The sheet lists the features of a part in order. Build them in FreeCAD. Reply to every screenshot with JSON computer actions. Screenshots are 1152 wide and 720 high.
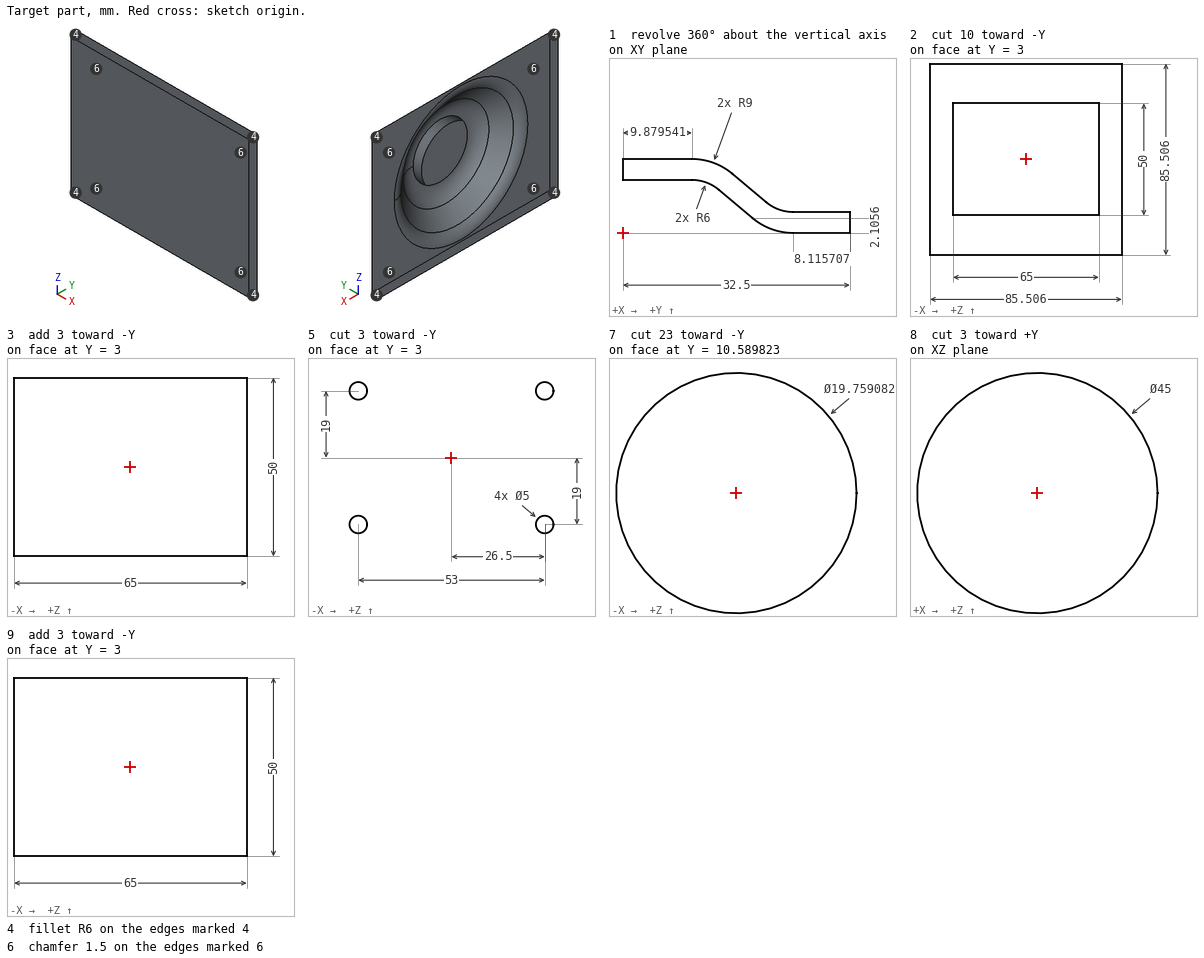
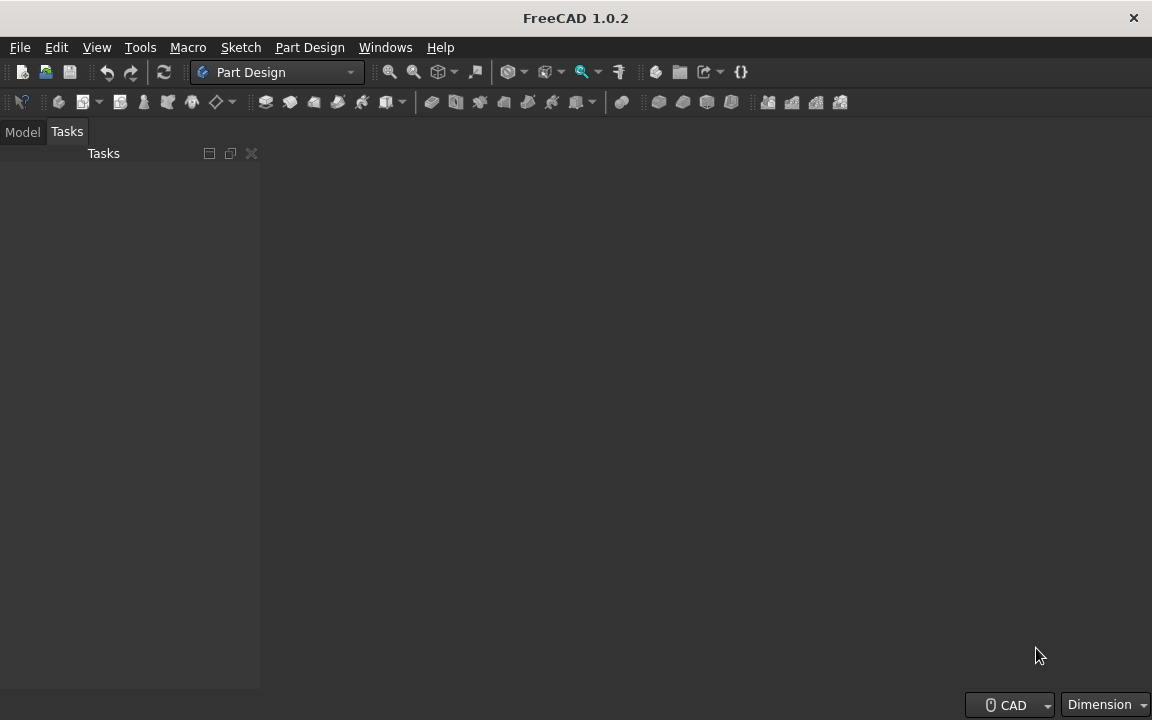
{"action": "left_click", "coordinate": [22, 72]}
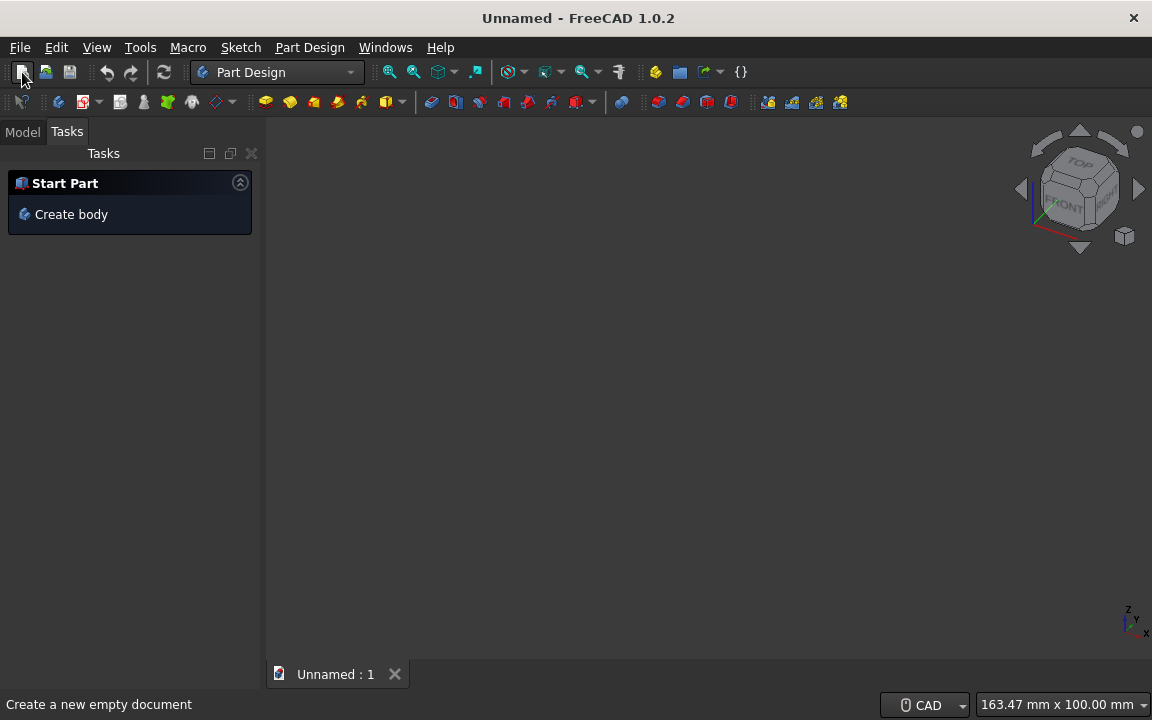
{"action": "left_click", "coordinate": [84, 102]}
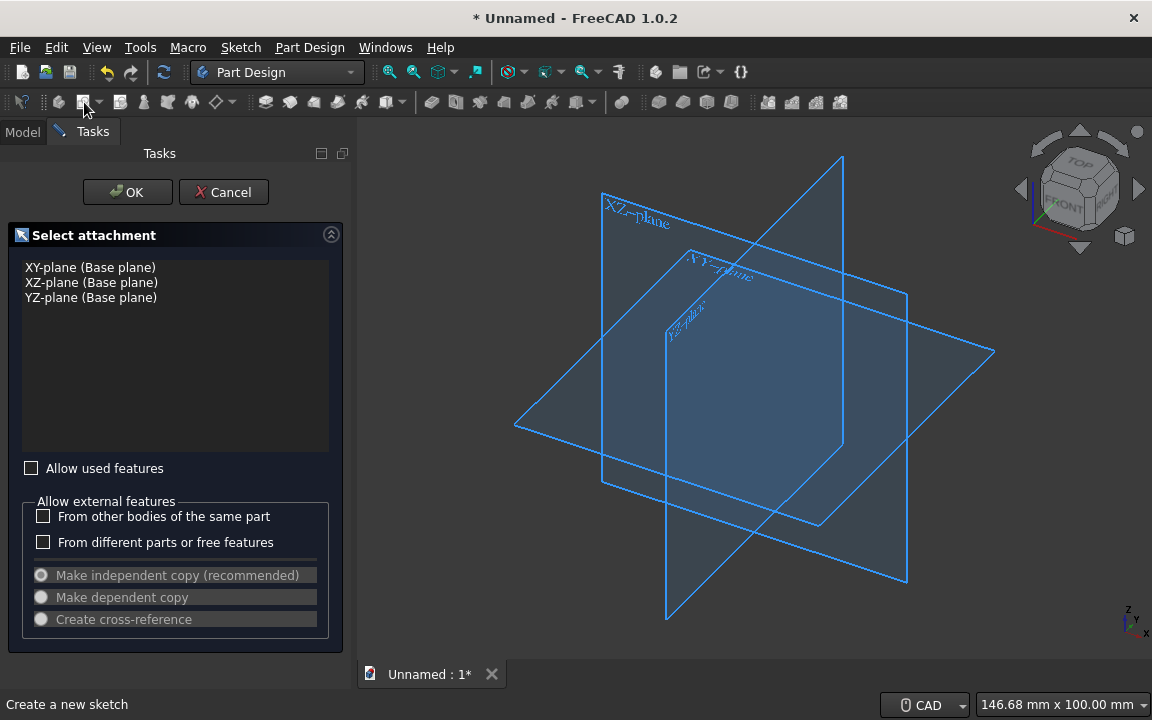
{"action": "left_click", "coordinate": [82, 268]}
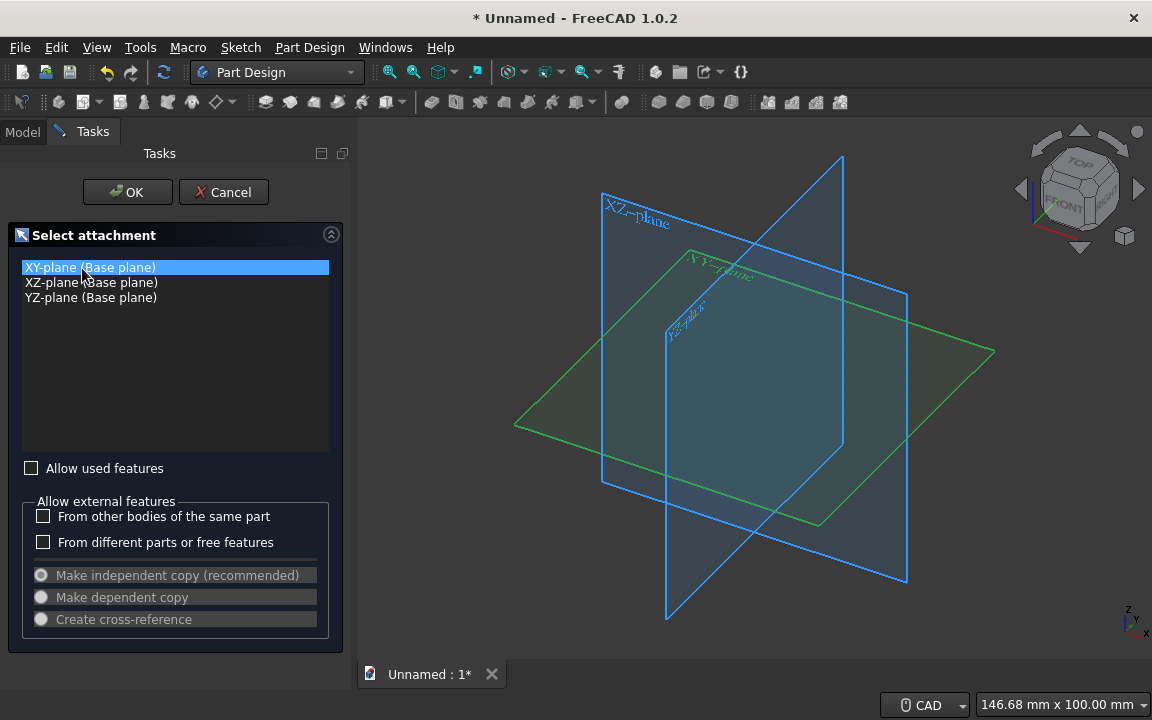
{"action": "left_click", "coordinate": [128, 192]}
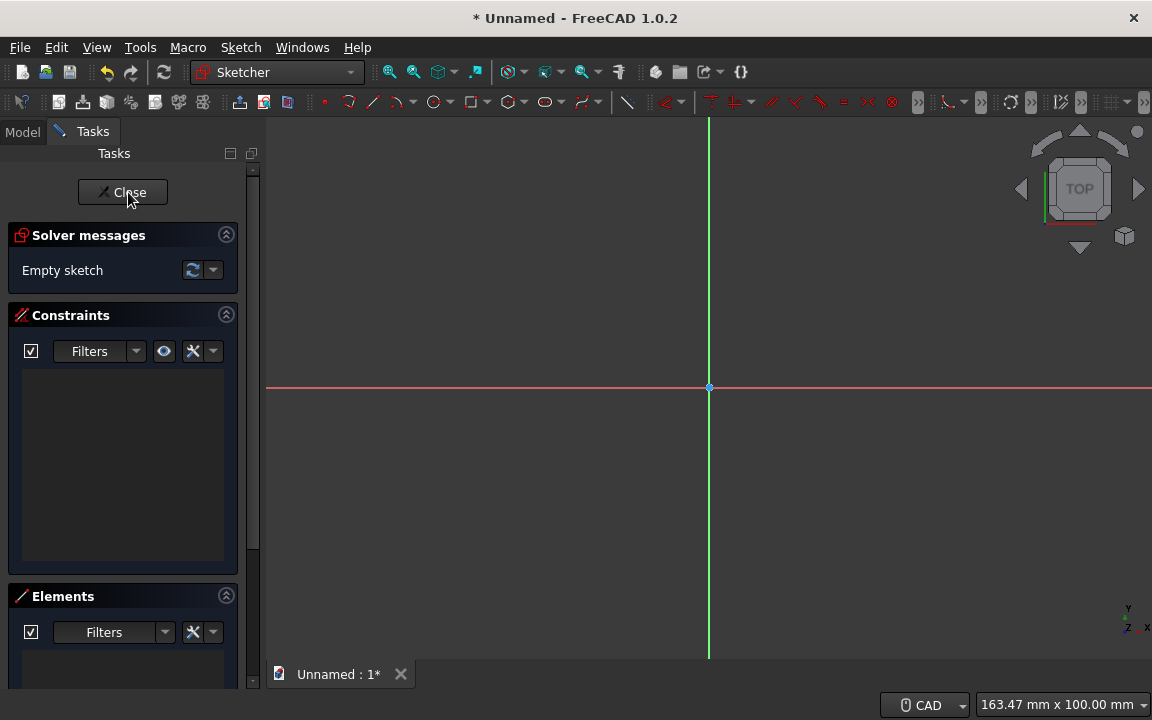
{"action": "scroll", "coordinate": [888, 343], "scroll_direction": "up", "scroll_amount": 5}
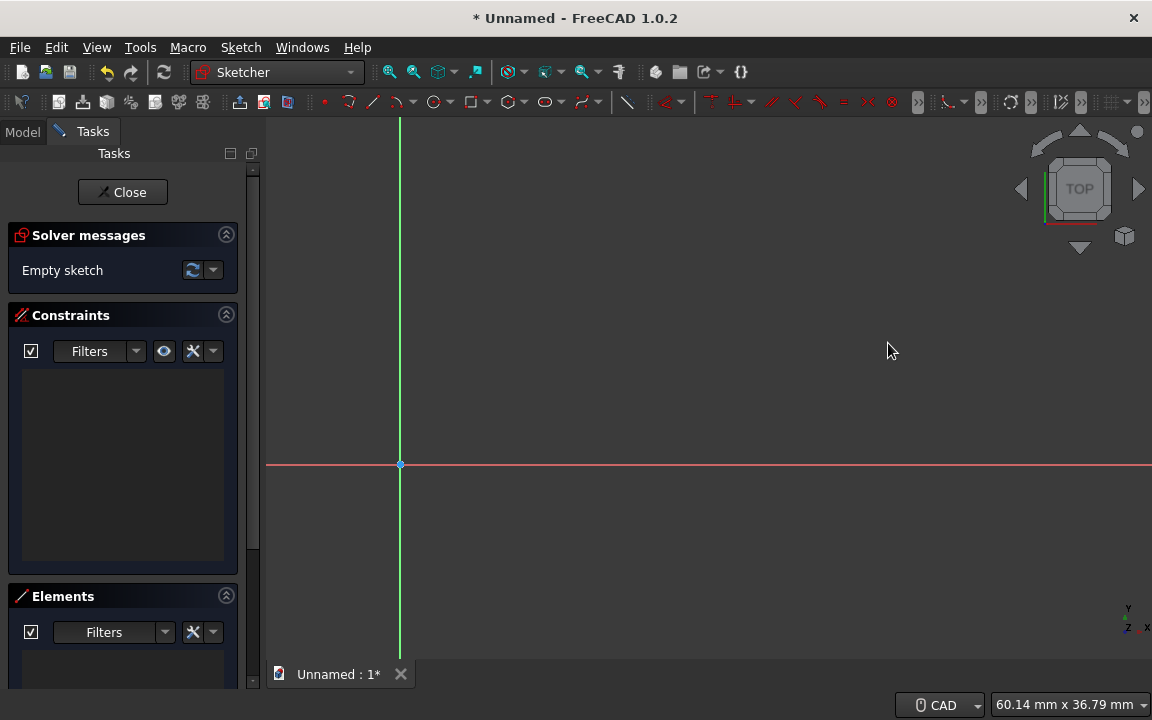
{"action": "left_click", "coordinate": [374, 102]}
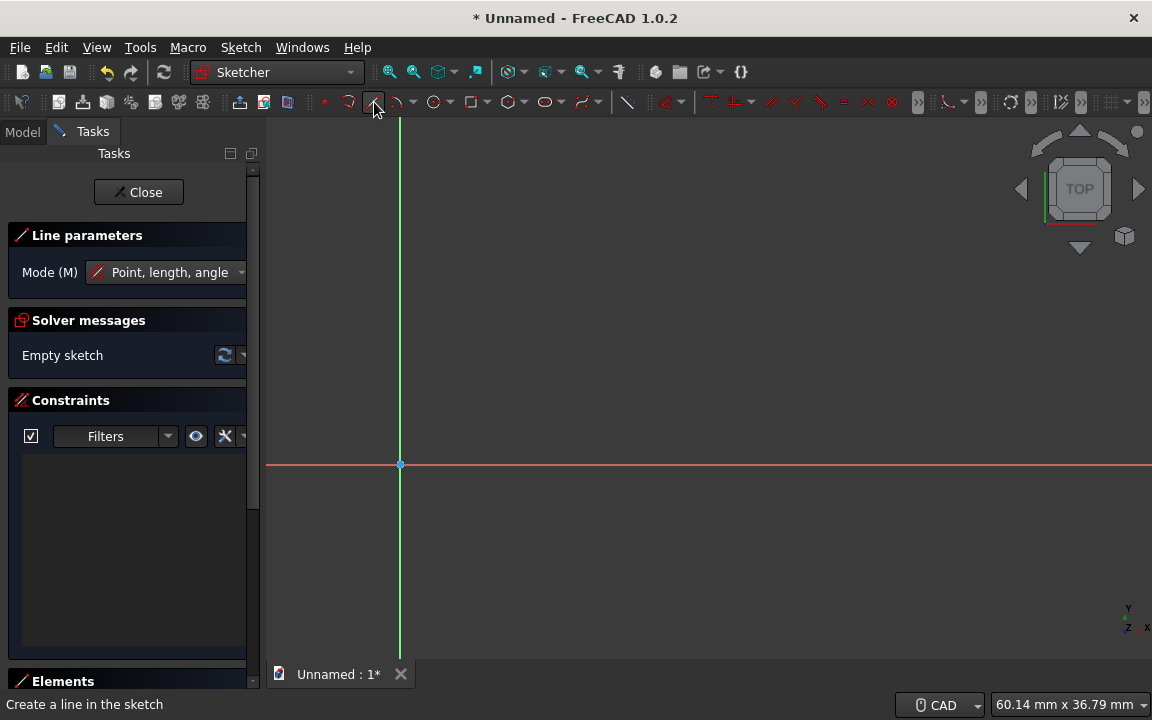
{"action": "left_click", "coordinate": [603, 373]}
{"action": "left_click", "coordinate": [674, 434]}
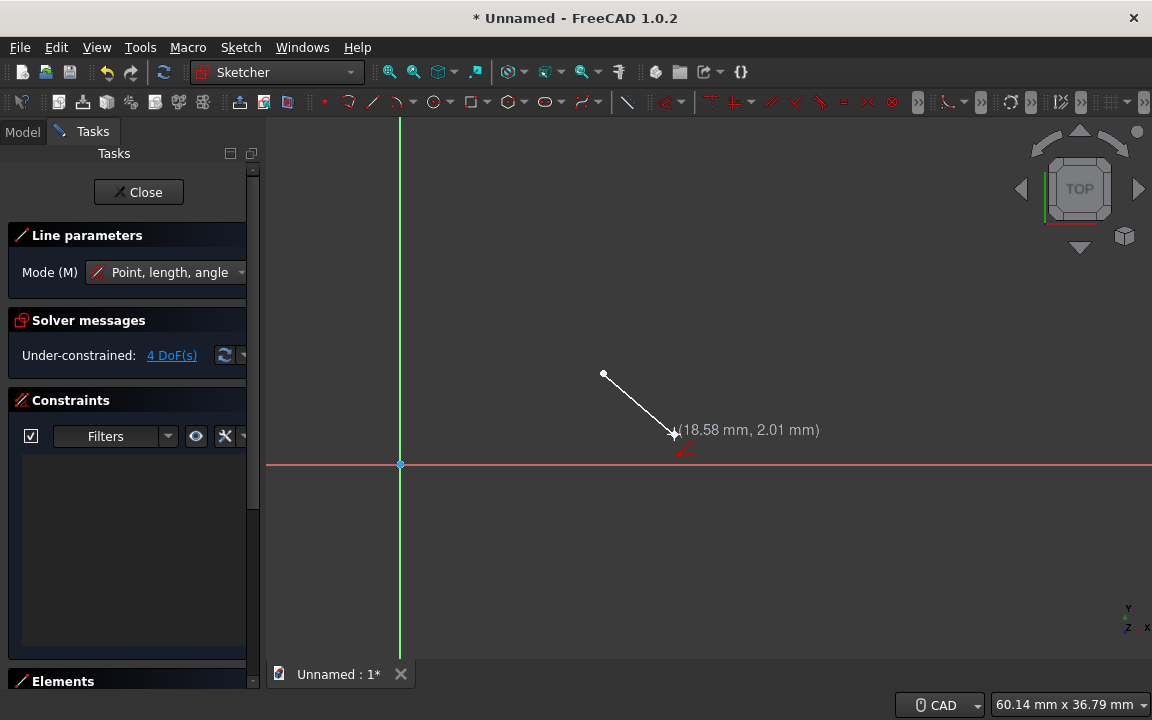
{"action": "left_click", "coordinate": [350, 102]}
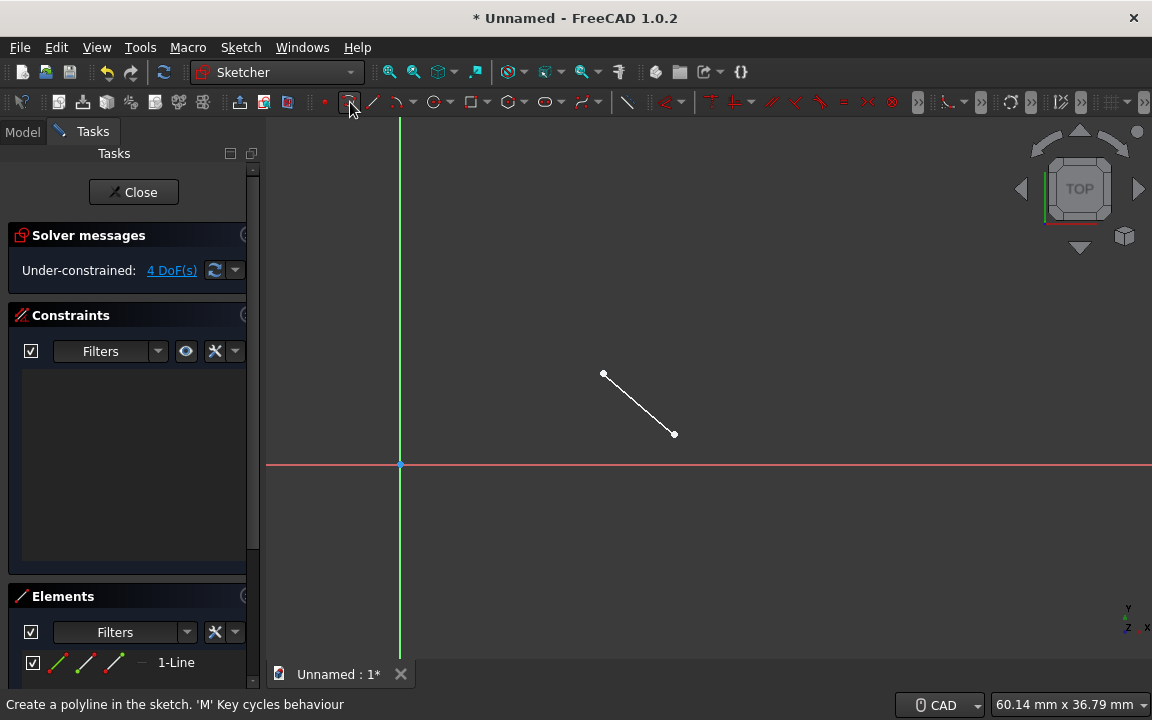
{"action": "left_click", "coordinate": [759, 465]}
{"action": "left_click", "coordinate": [879, 456]}
{"action": "left_click", "coordinate": [879, 420]}
{"action": "left_click", "coordinate": [759, 420]}
{"action": "right_click", "coordinate": [759, 420]}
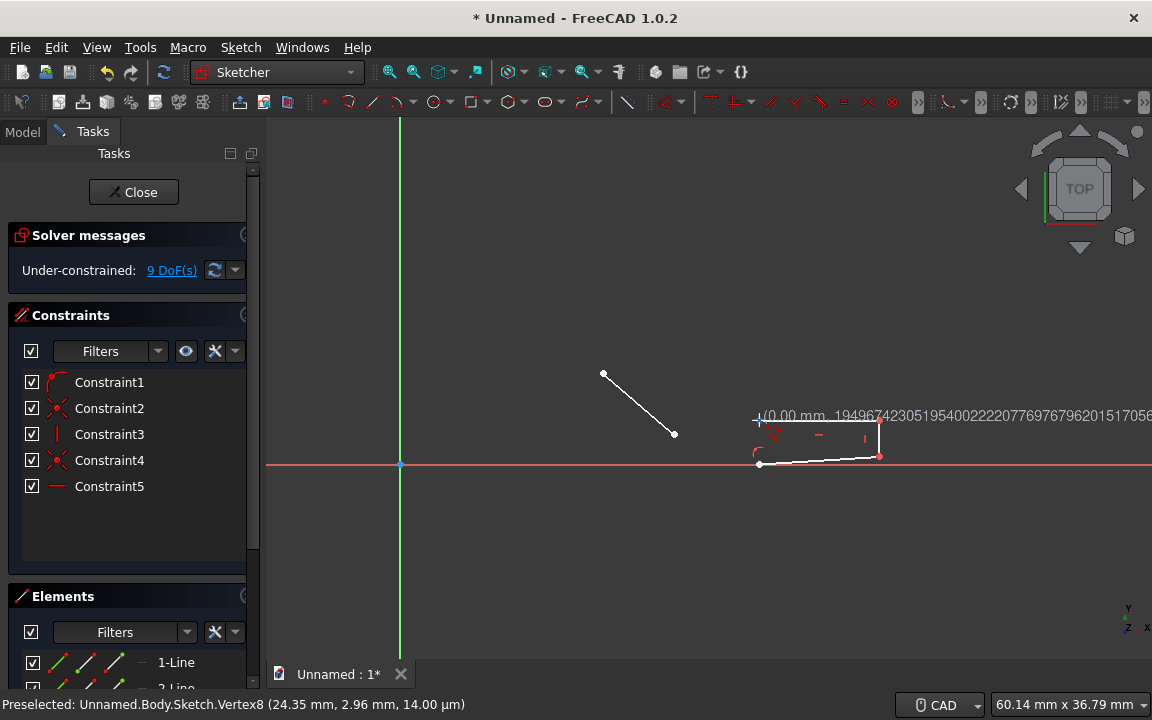
{"action": "left_click", "coordinate": [374, 102]}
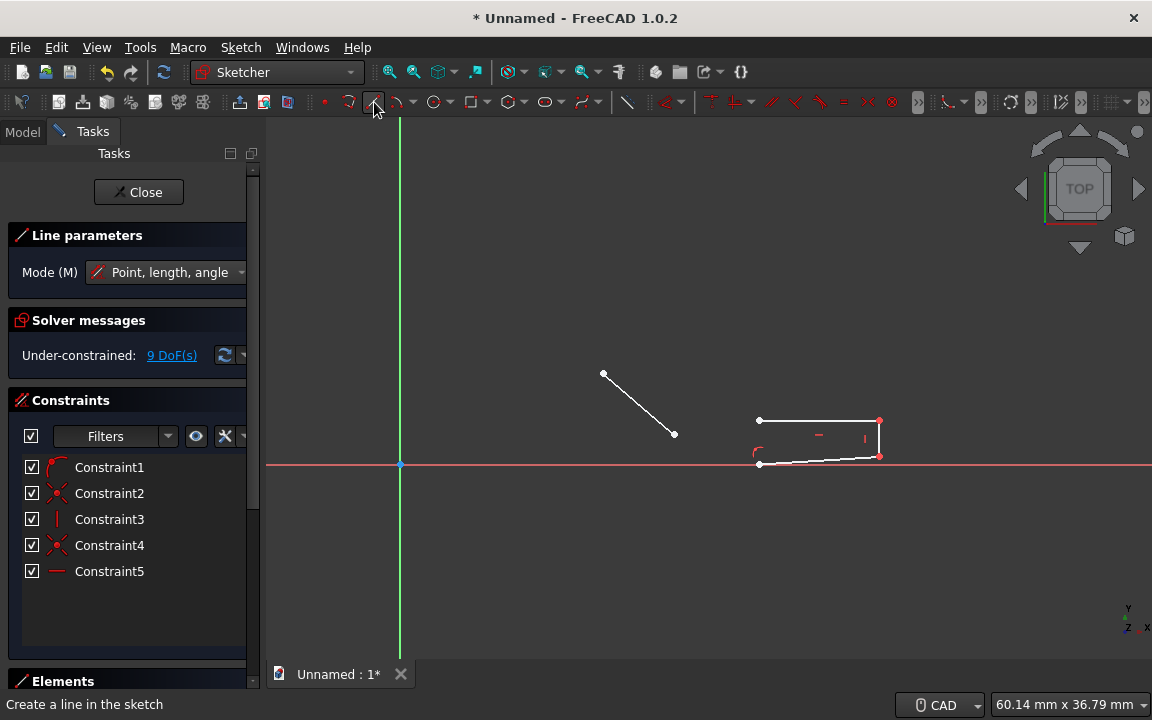
{"action": "left_click", "coordinate": [703, 400]}
{"action": "left_click", "coordinate": [631, 340]}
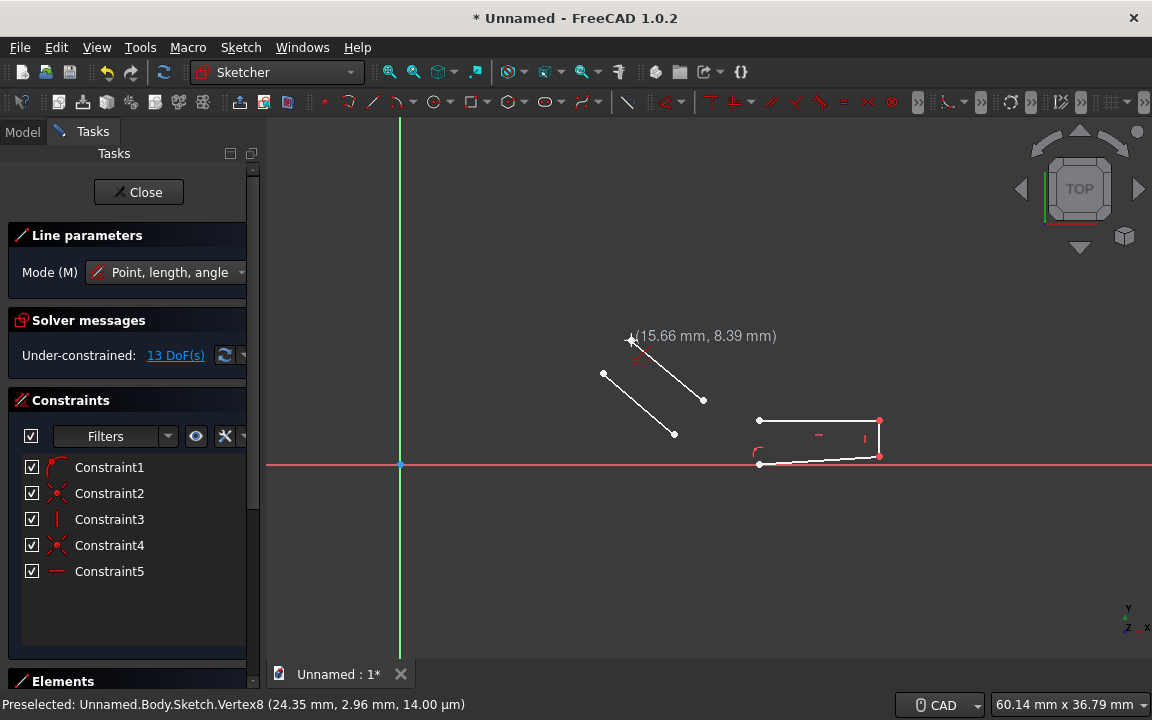
{"action": "left_click", "coordinate": [350, 102]}